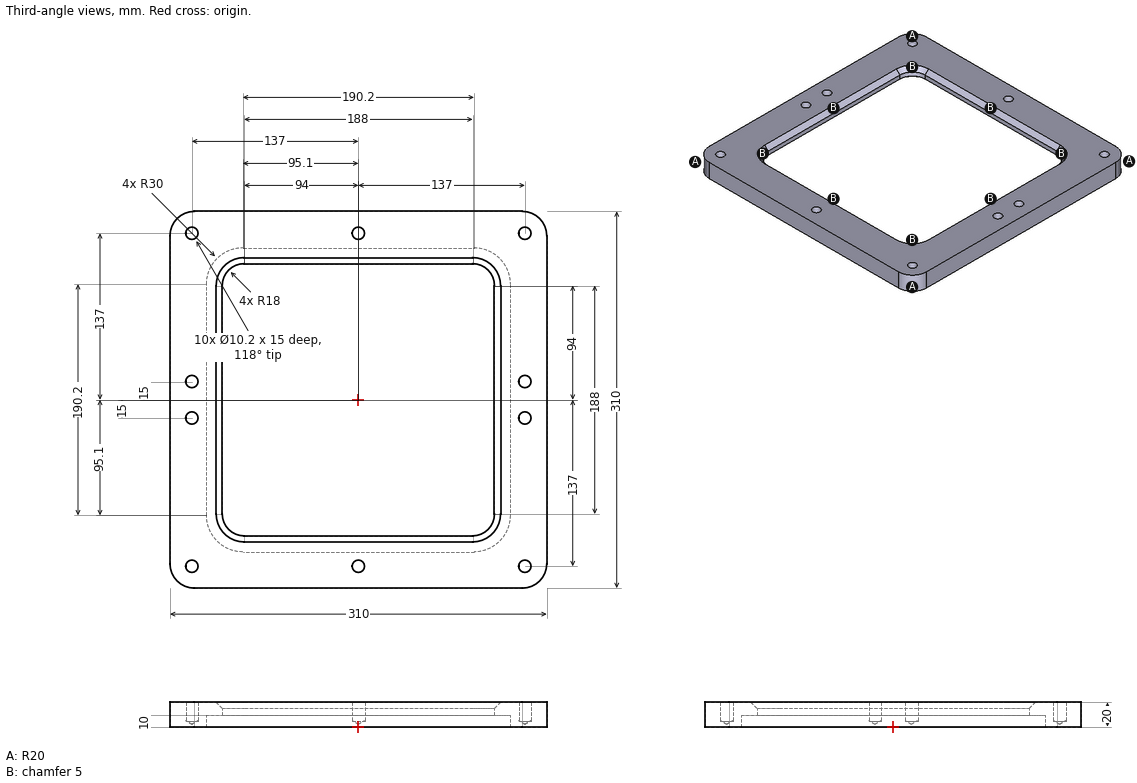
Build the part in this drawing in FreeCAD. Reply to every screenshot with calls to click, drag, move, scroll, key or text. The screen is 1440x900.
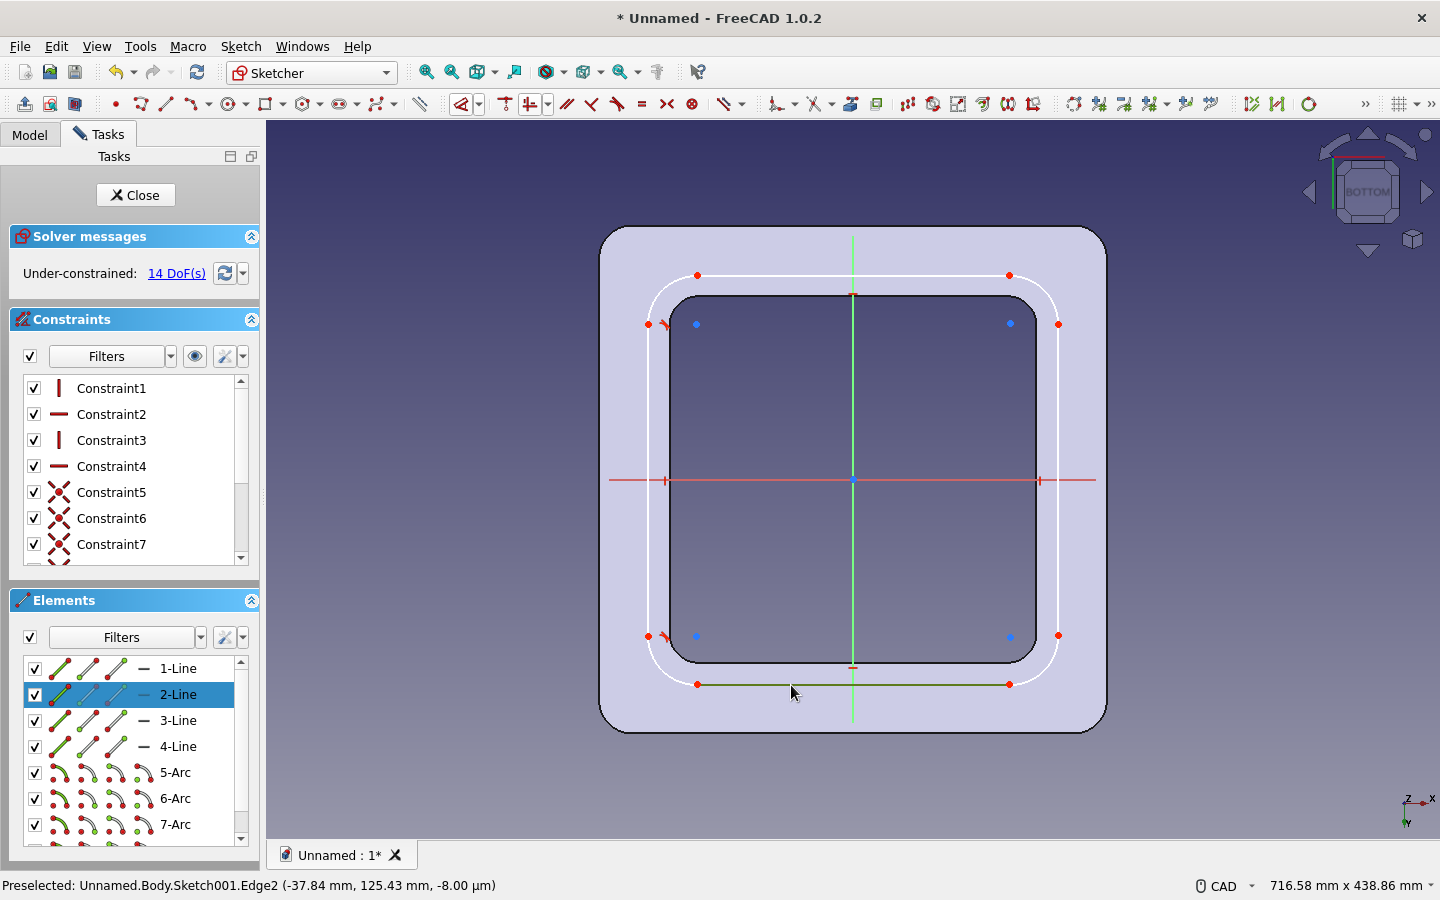
click(653, 658)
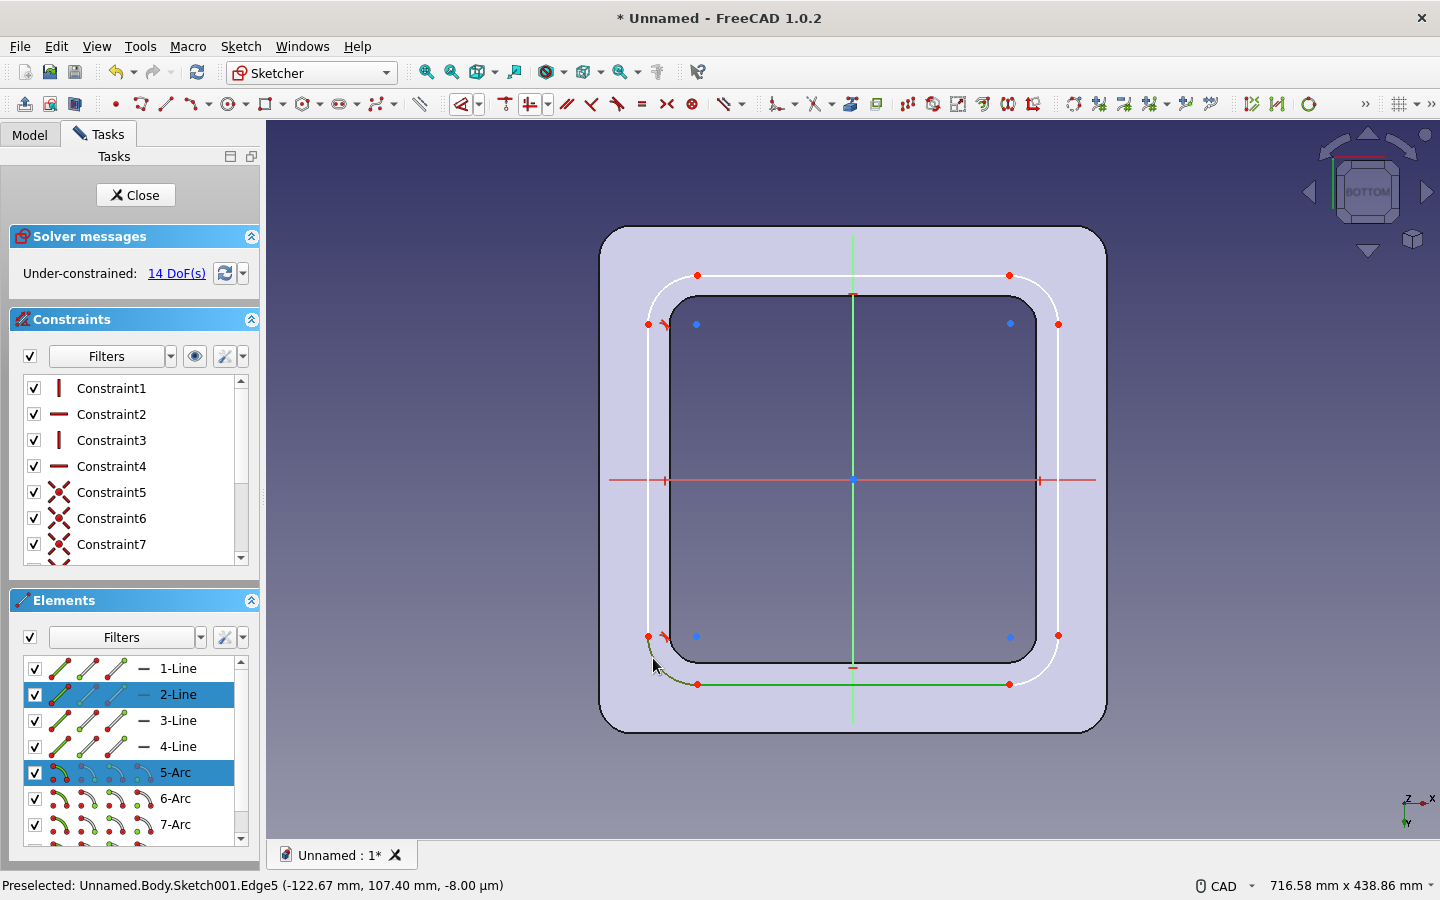
click(617, 104)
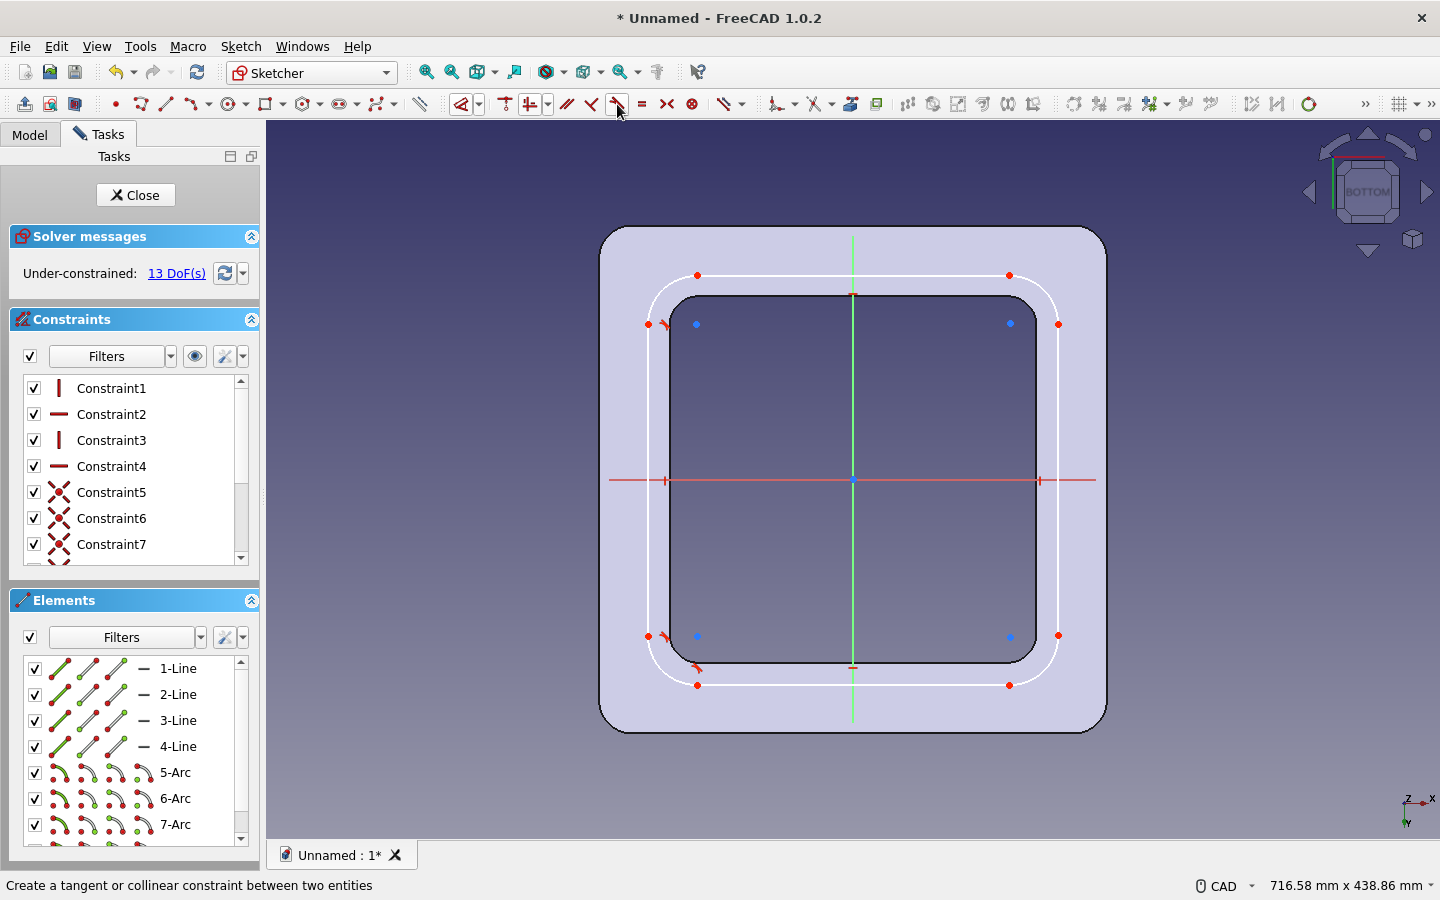
click(791, 685)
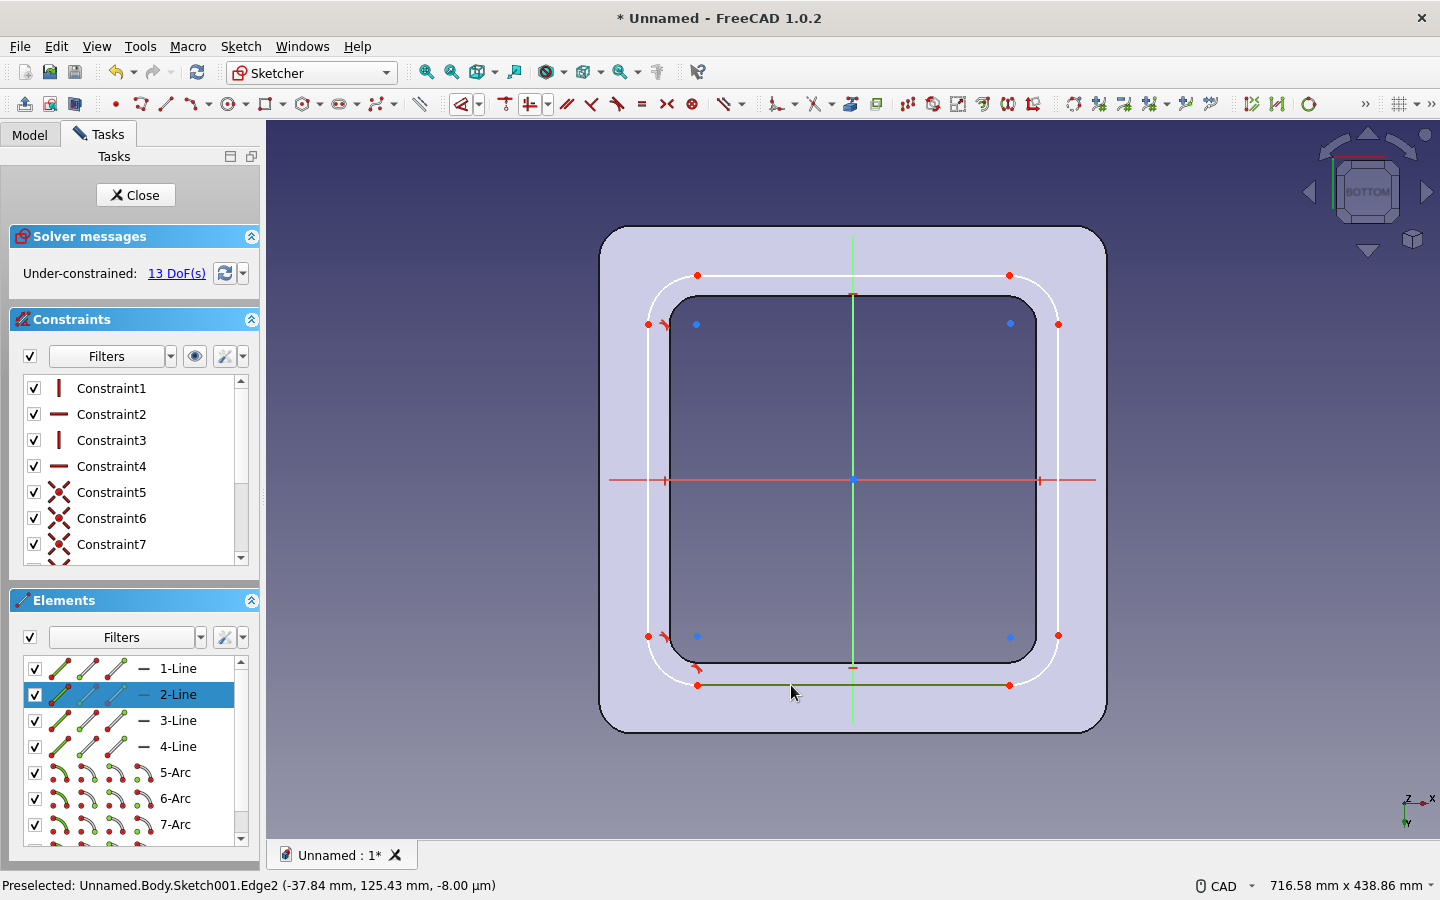
click(1031, 680)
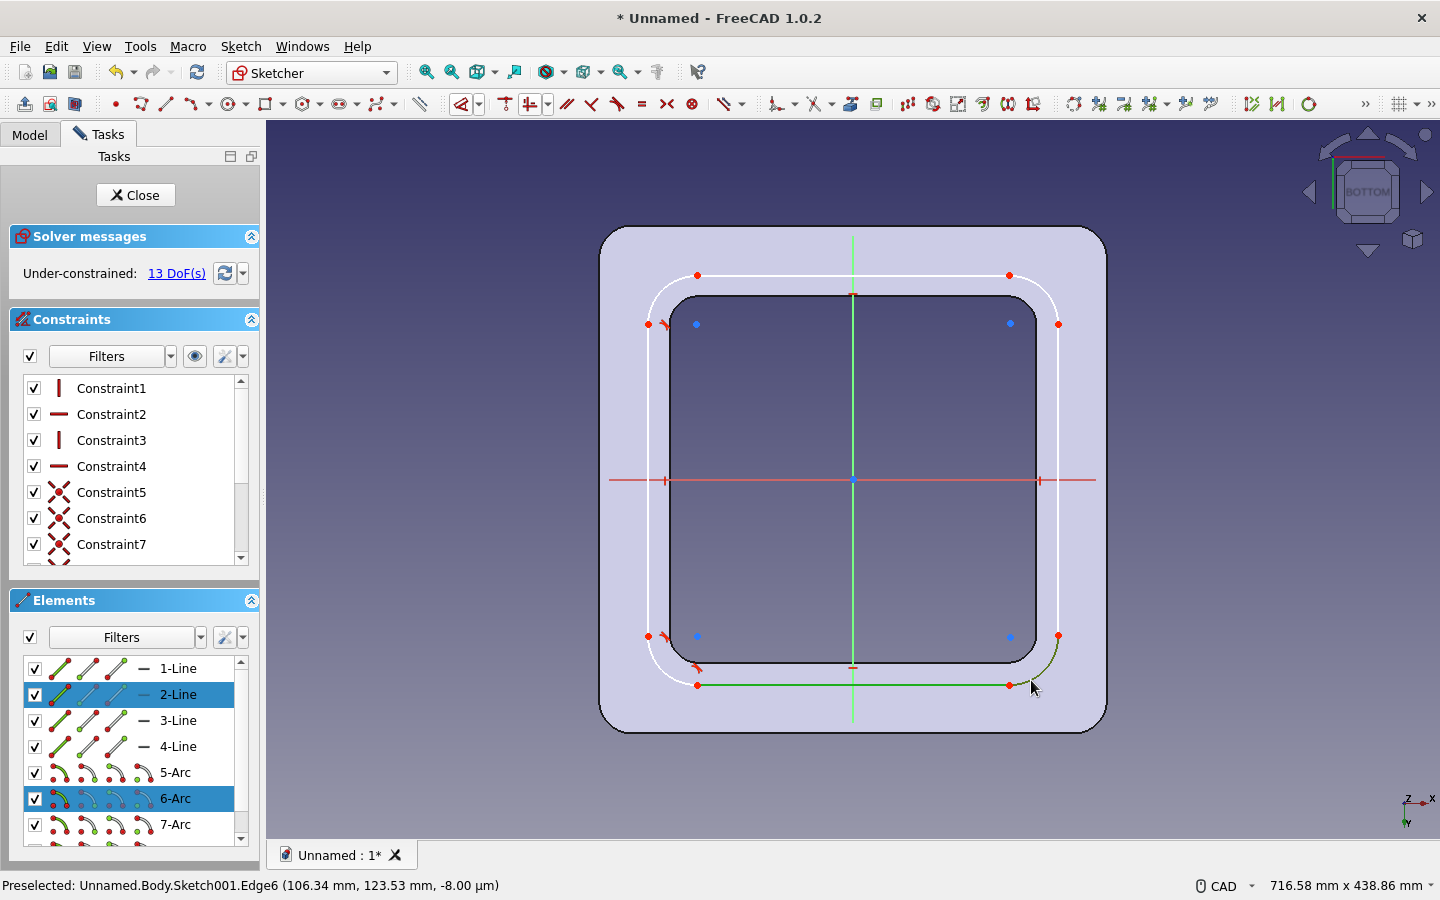
click(617, 104)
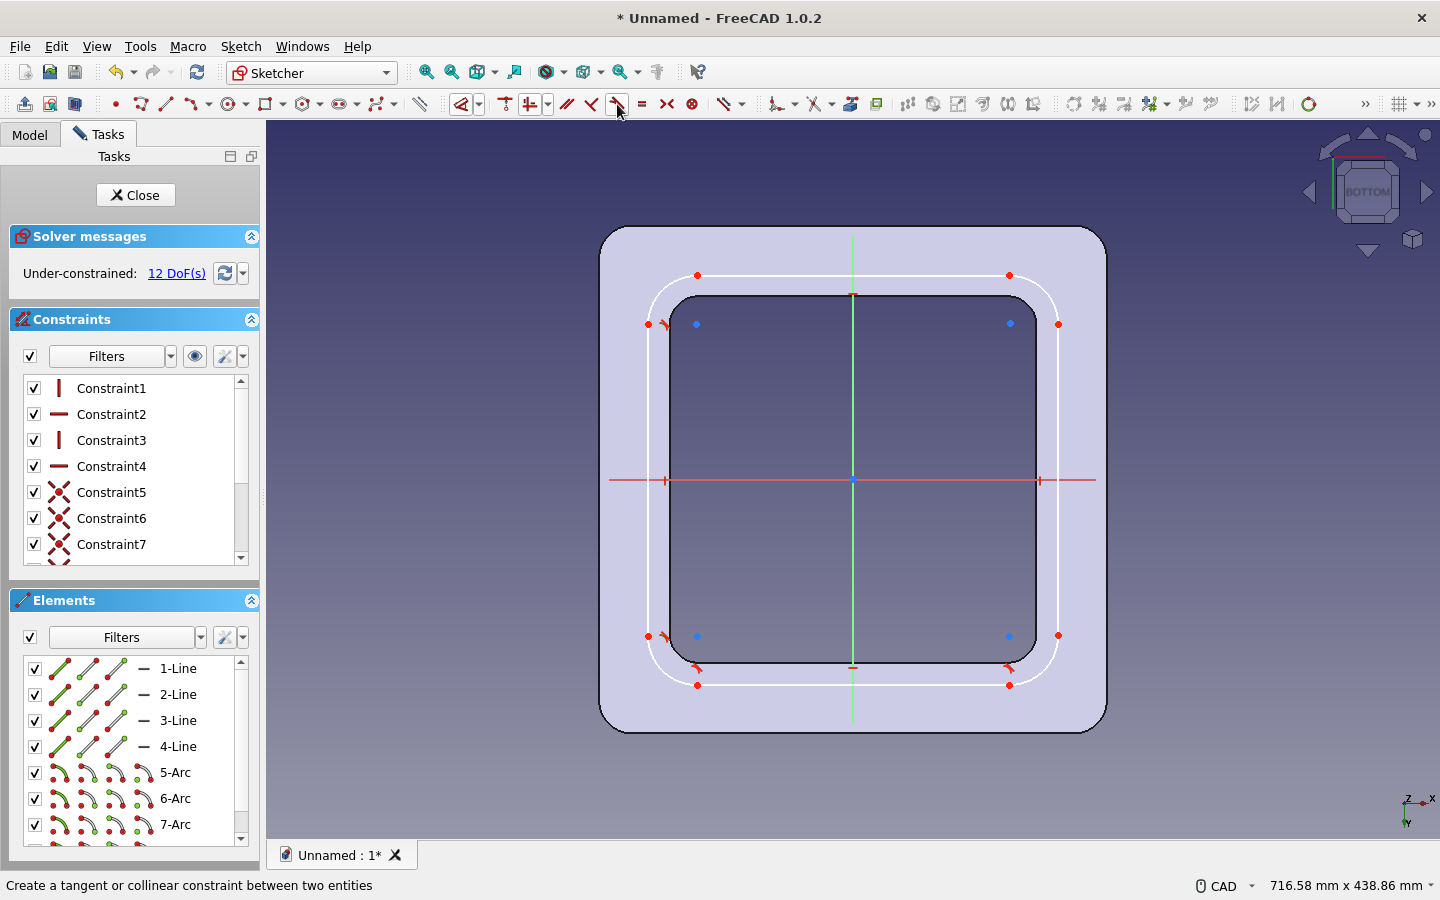
click(1058, 543)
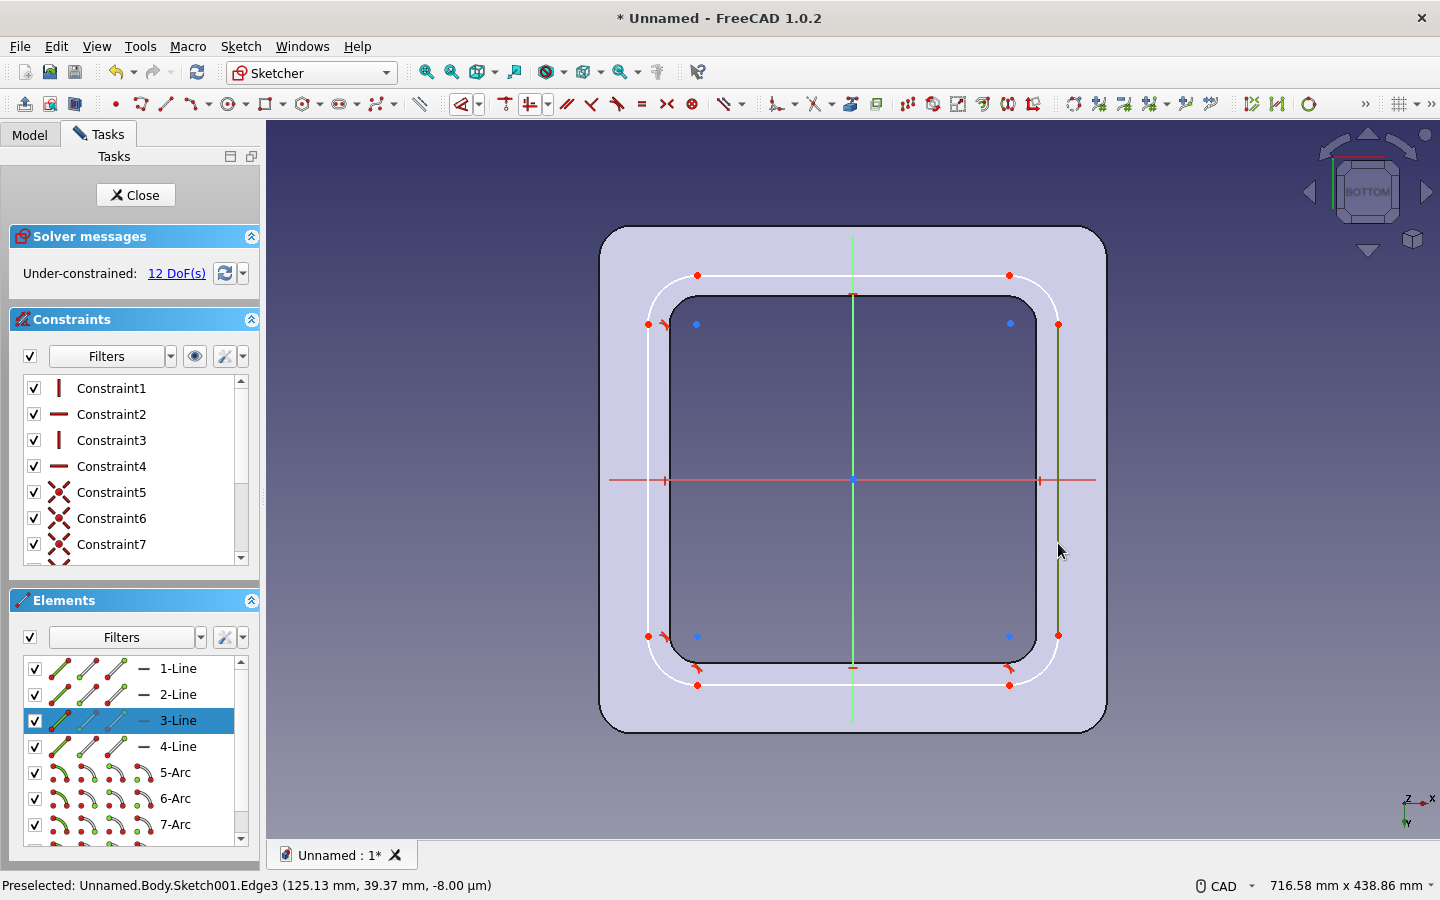
click(1031, 680)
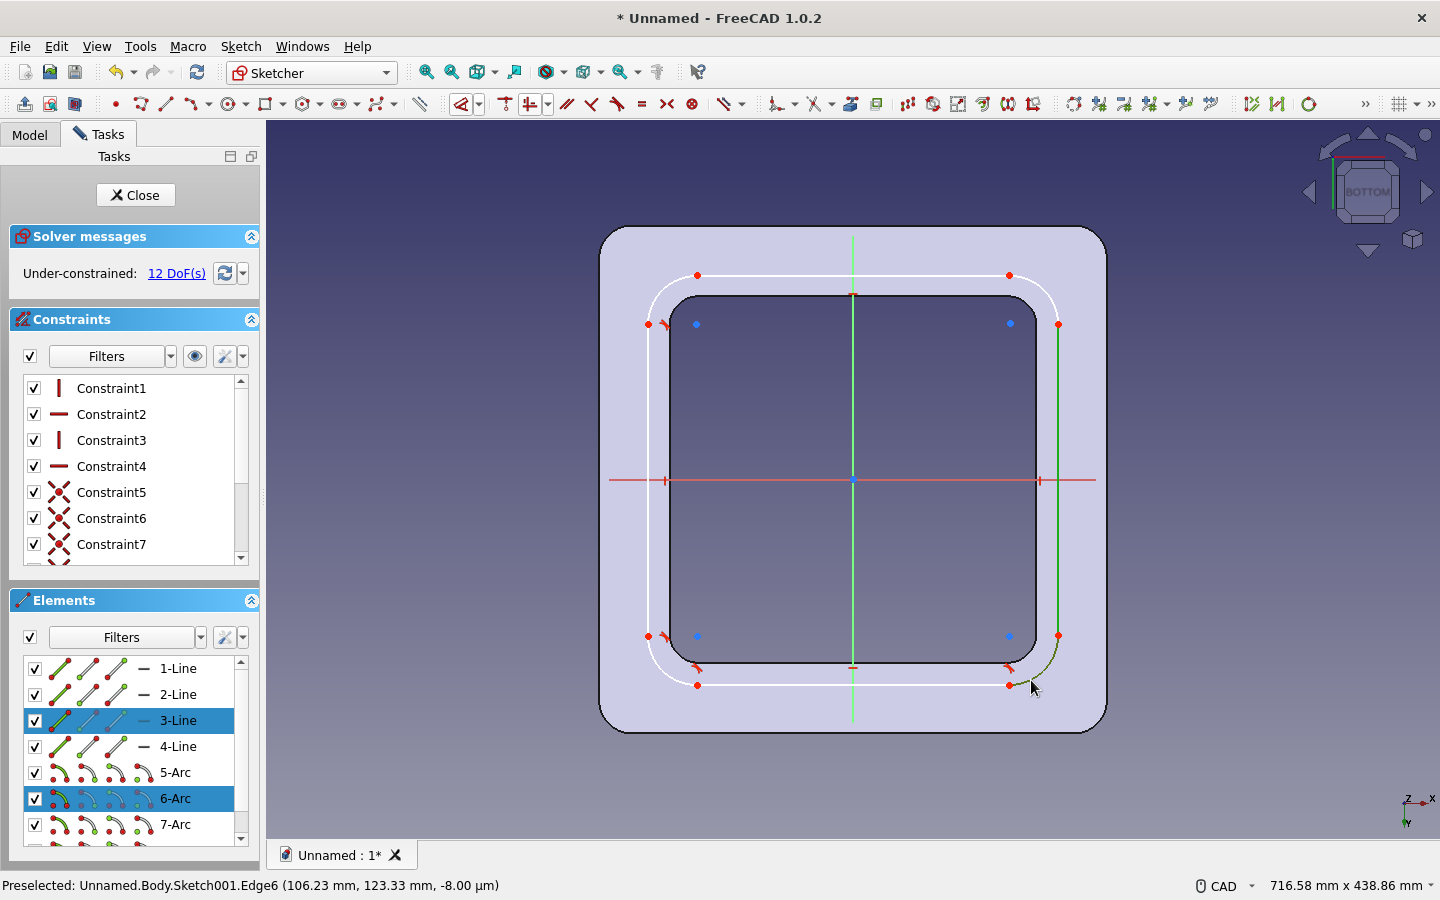
click(617, 104)